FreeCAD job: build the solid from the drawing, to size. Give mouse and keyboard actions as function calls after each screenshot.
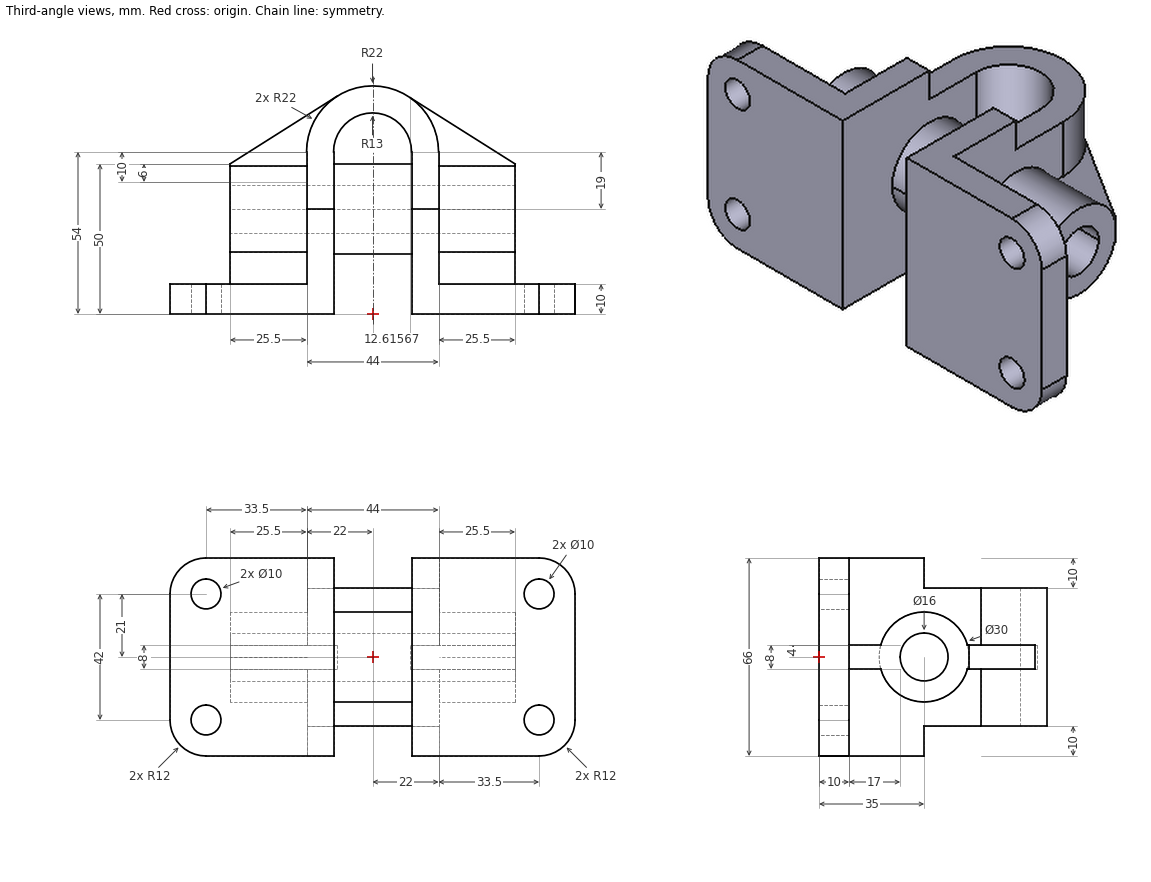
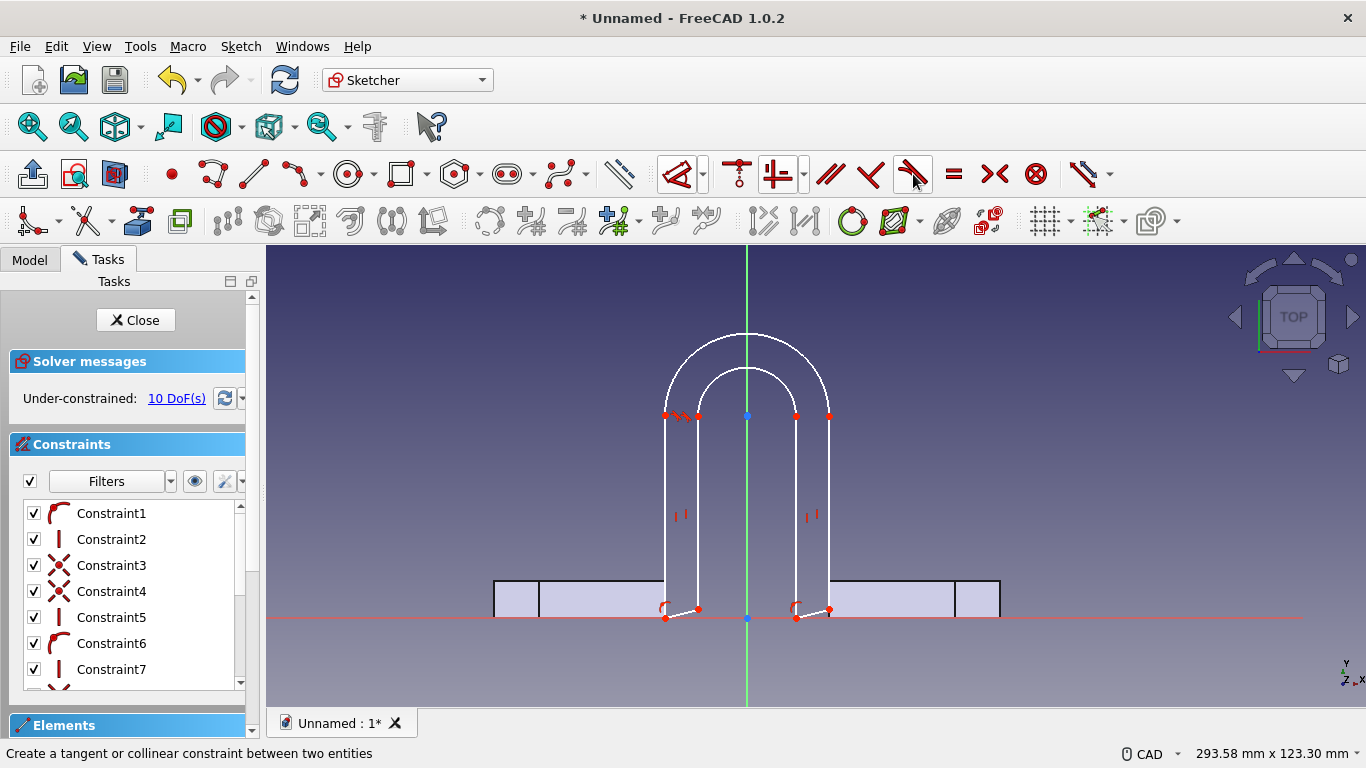
click(796, 477)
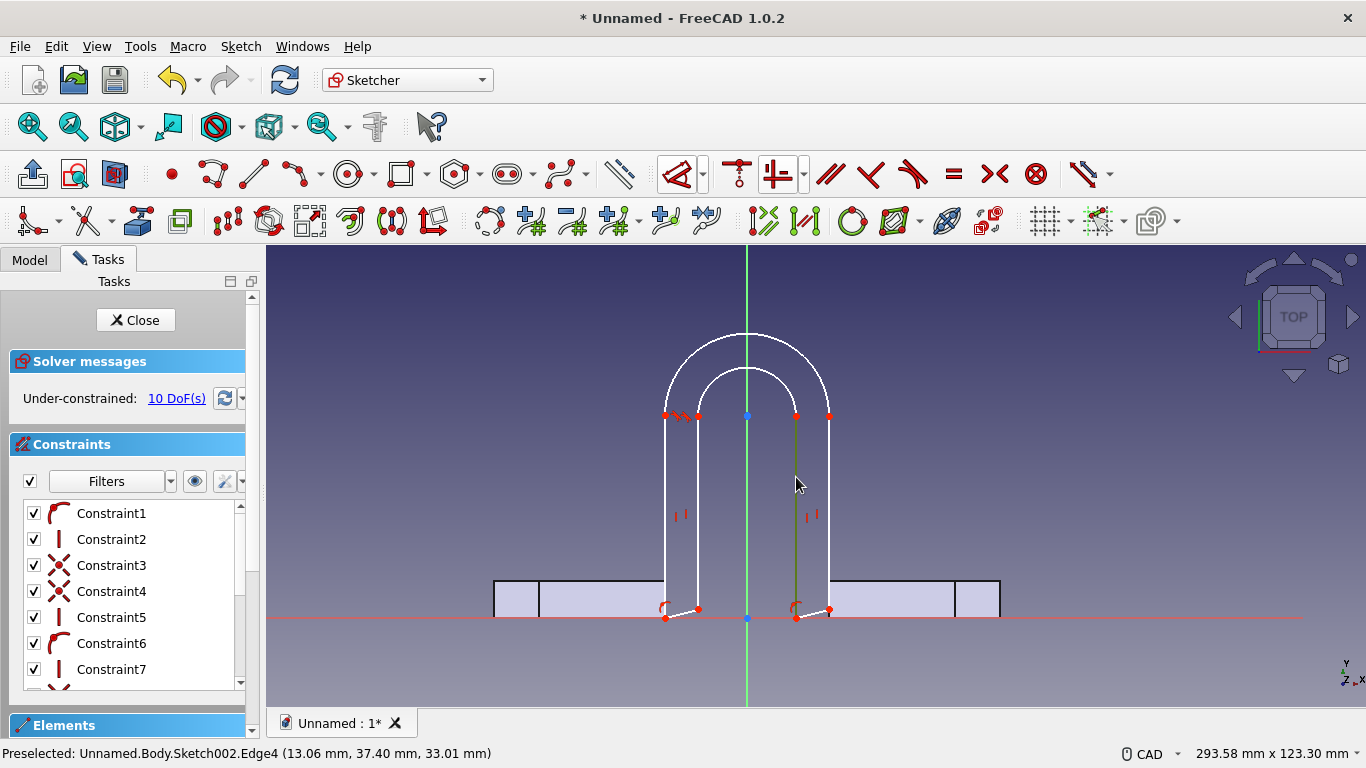
click(776, 377)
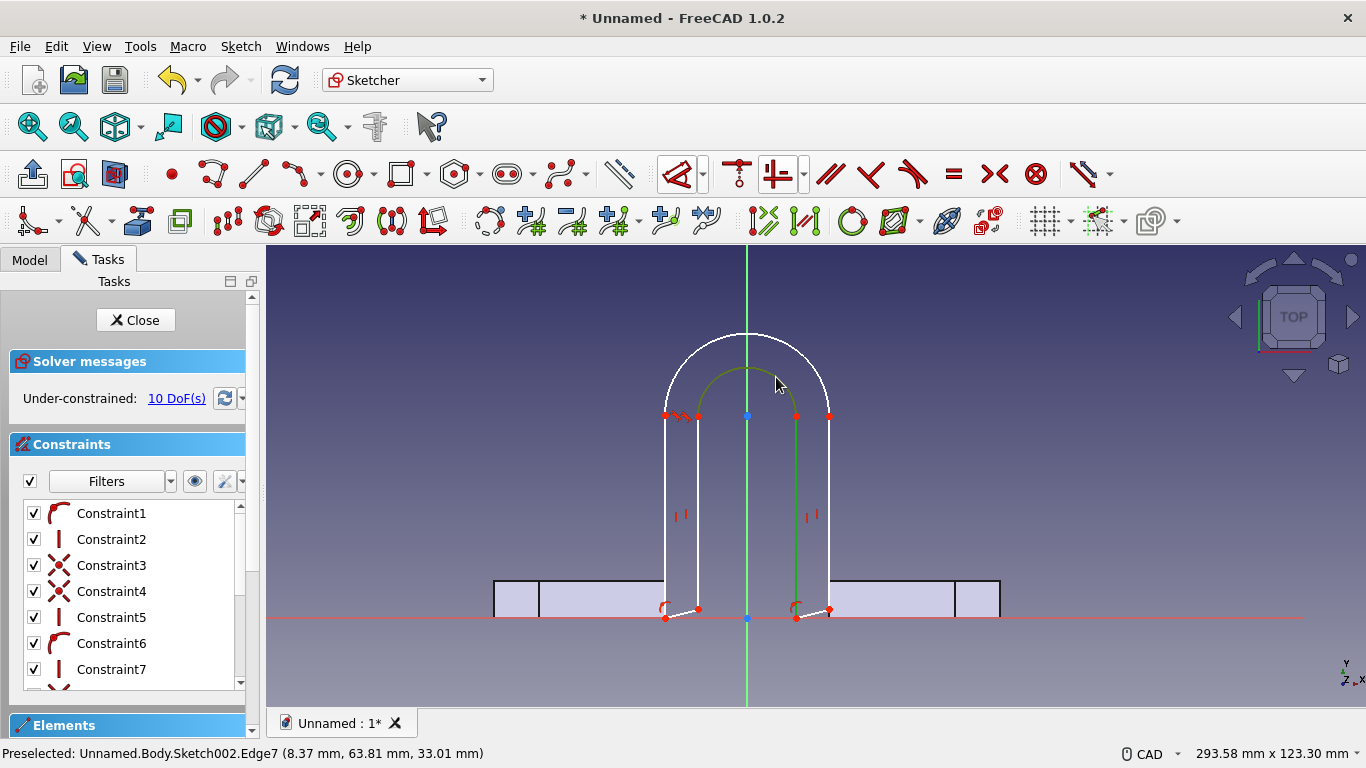
click(913, 174)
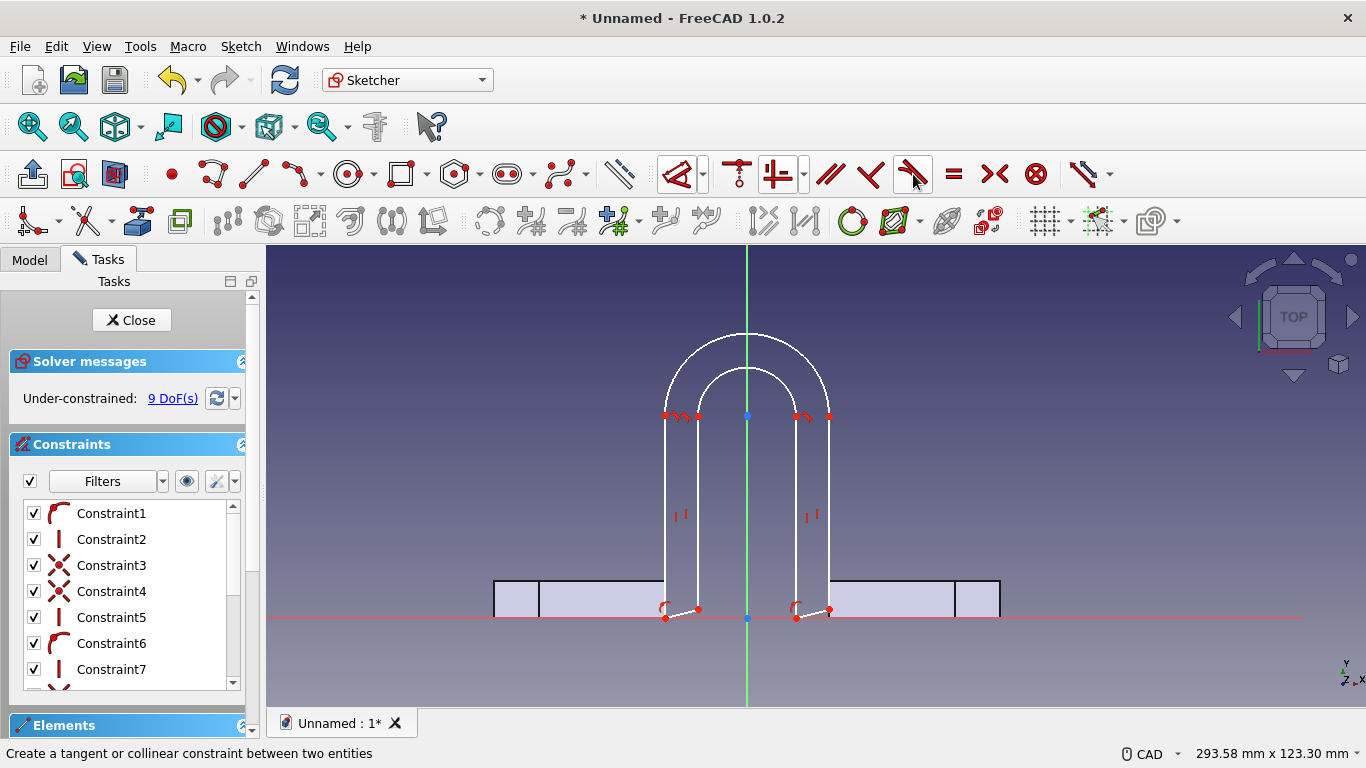
click(829, 552)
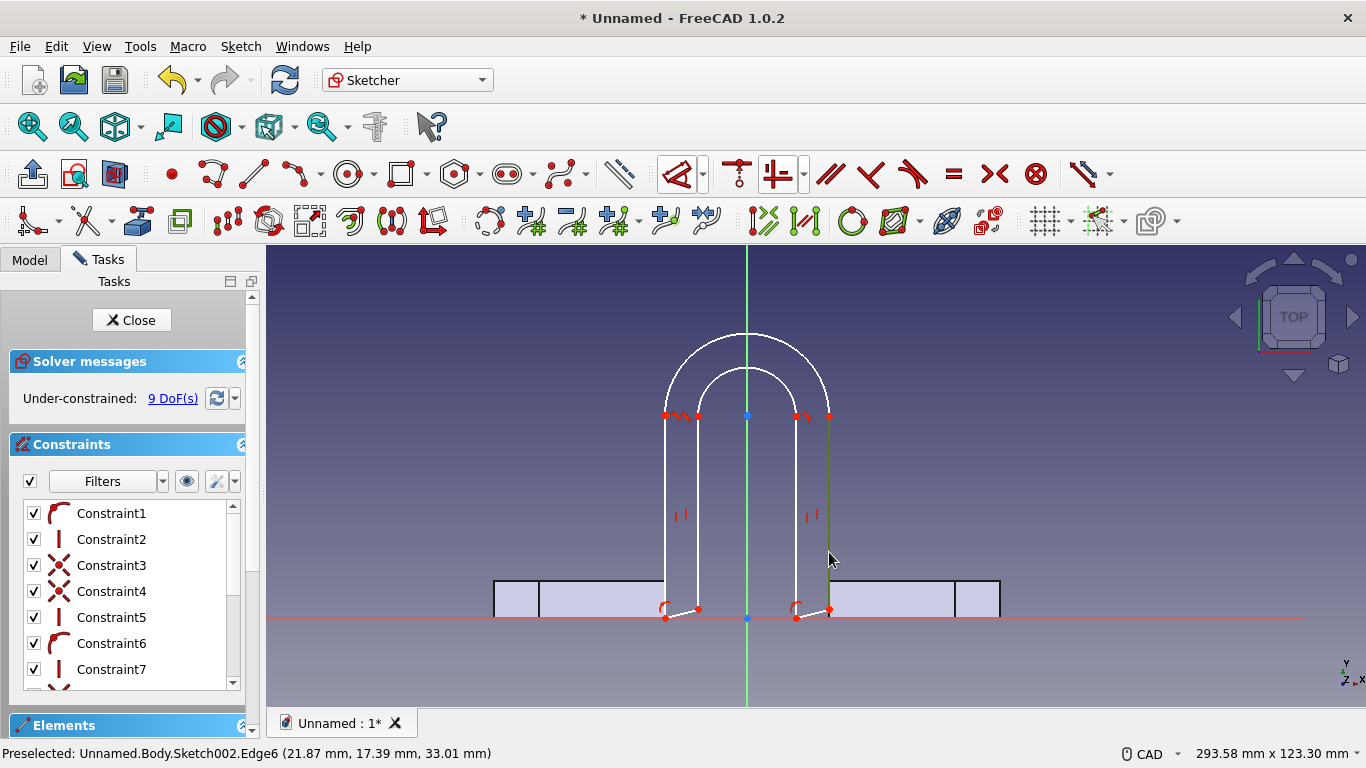
click(796, 350)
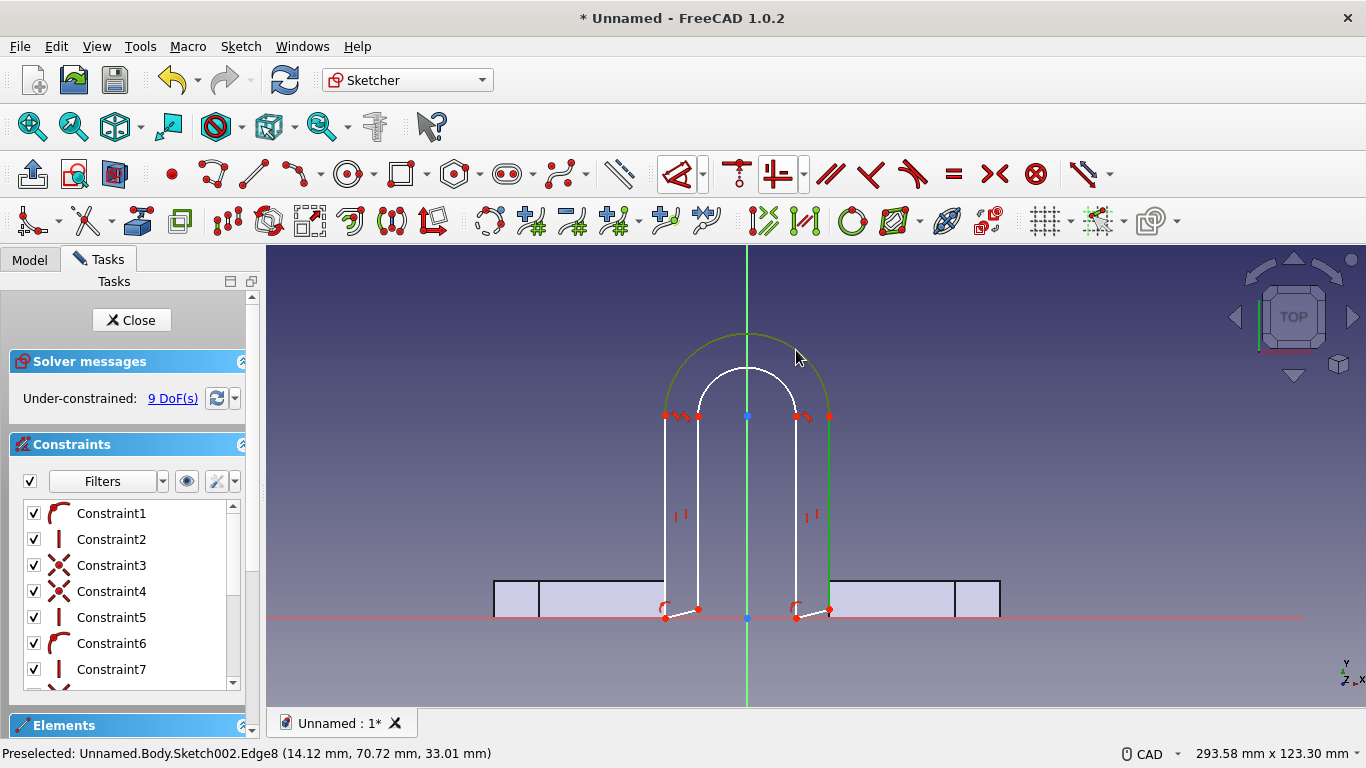
click(913, 174)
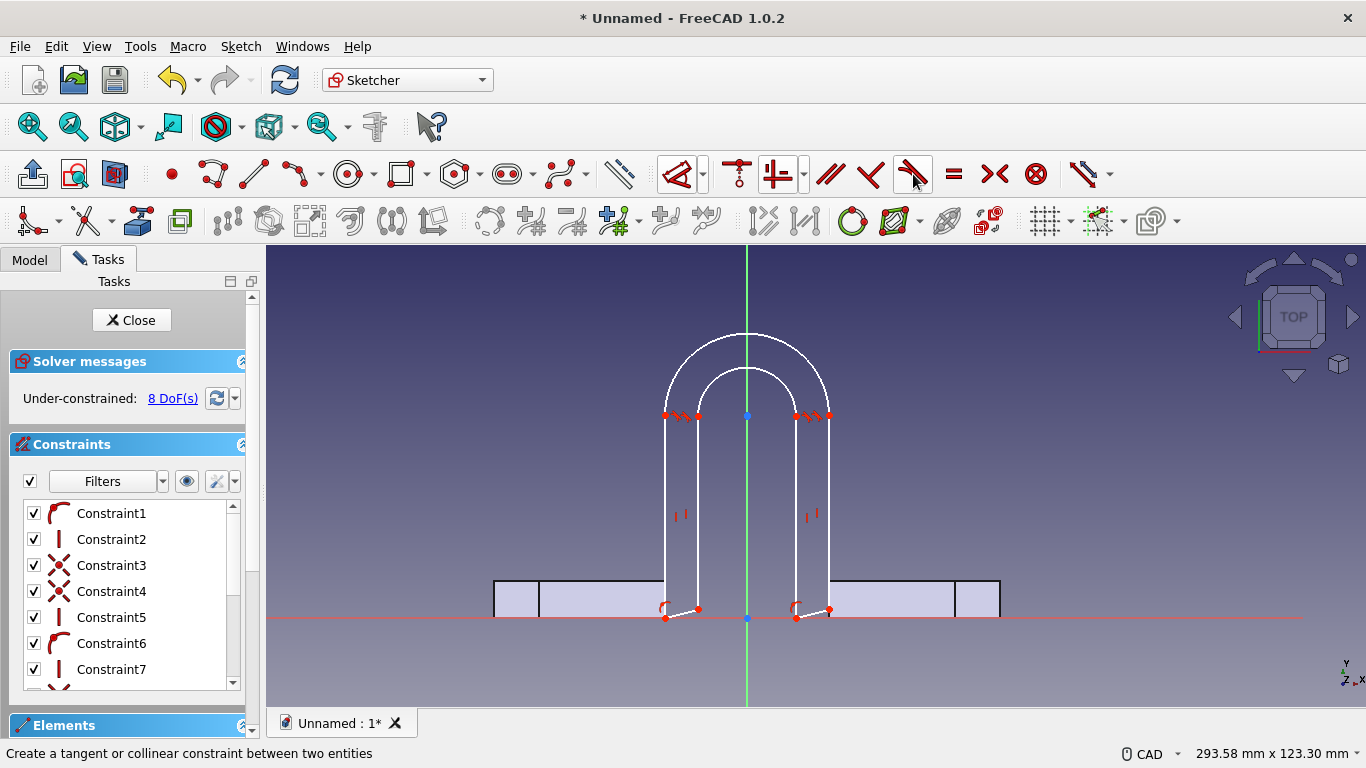
scroll(675, 616, up, 2)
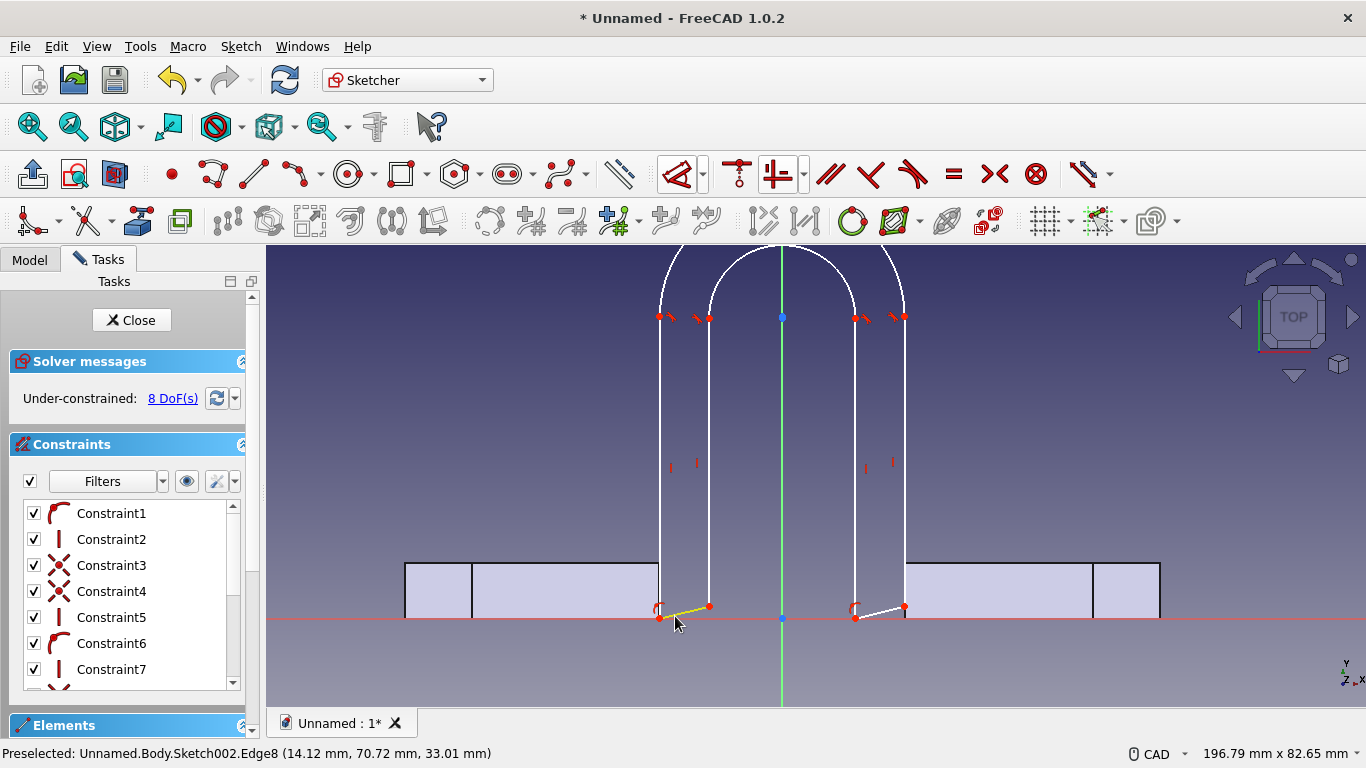
click(675, 615)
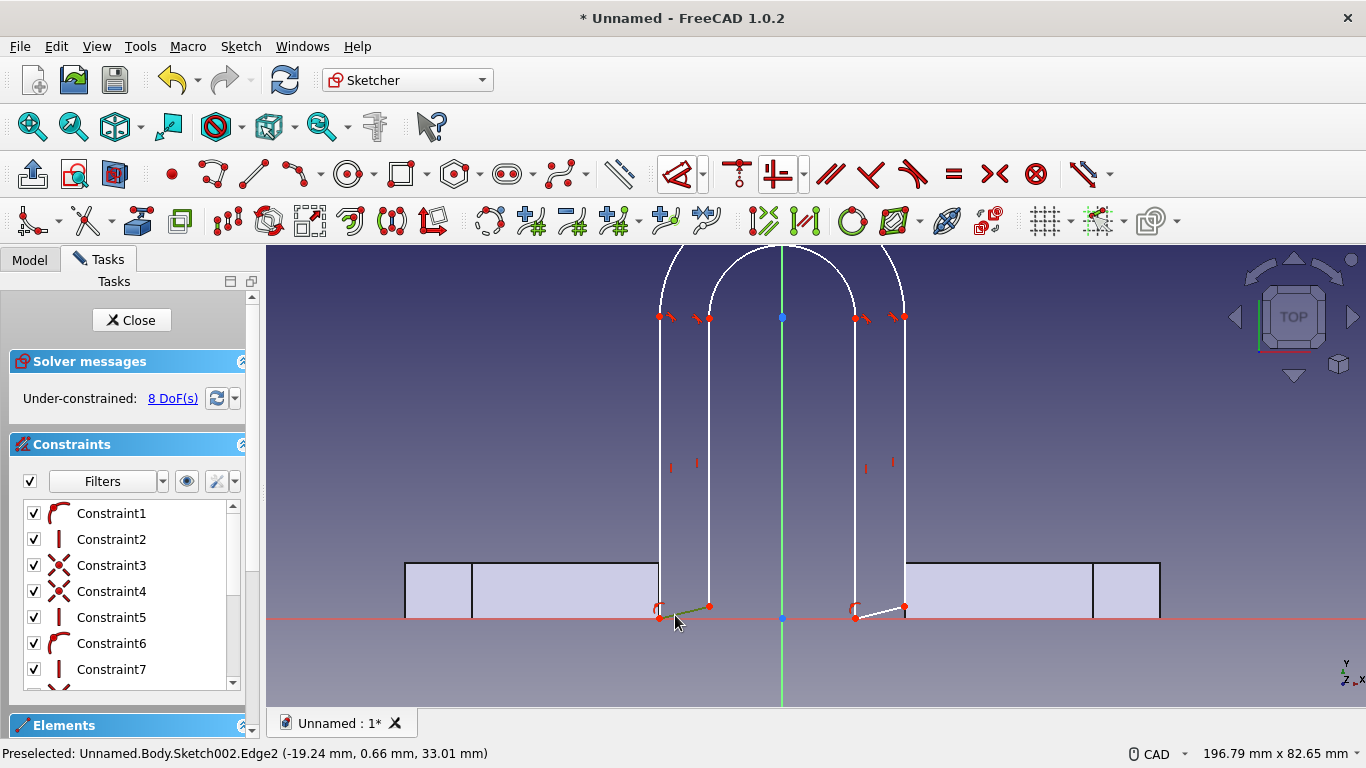
click(804, 174)